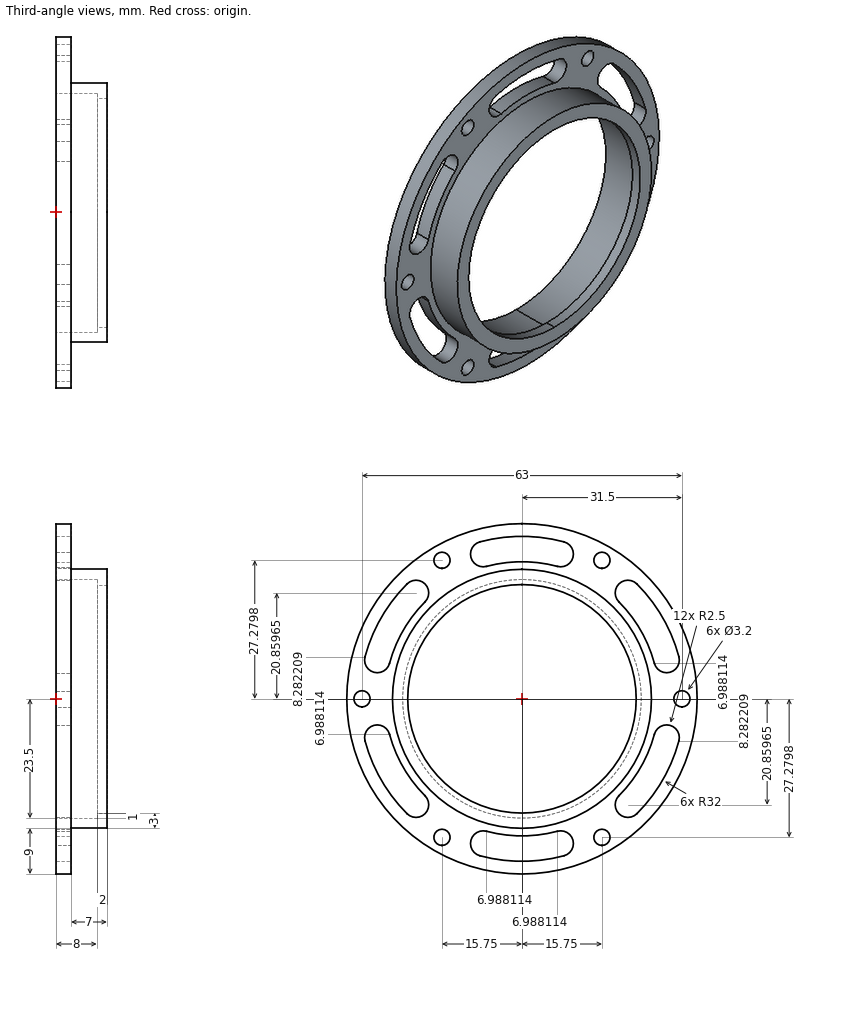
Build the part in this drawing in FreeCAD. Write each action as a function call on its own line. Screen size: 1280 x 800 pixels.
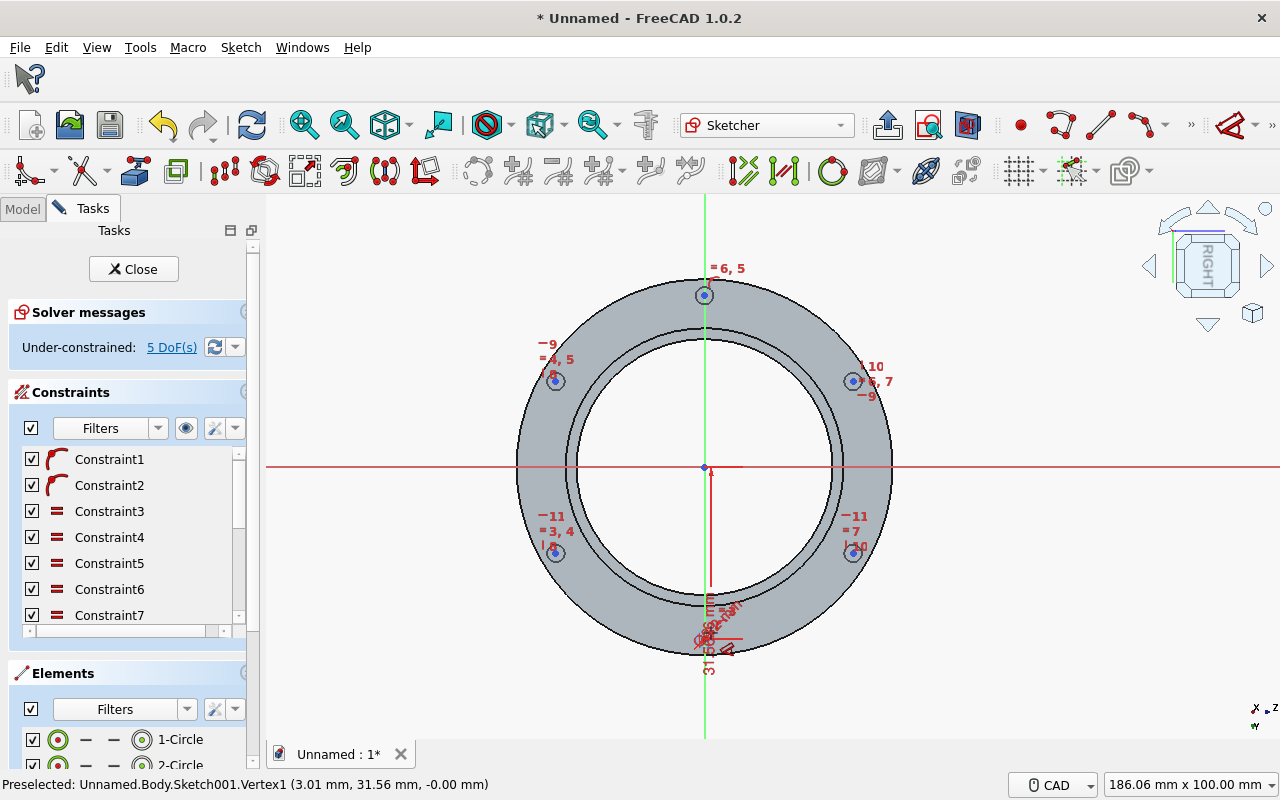
click(705, 296)
click(739, 388)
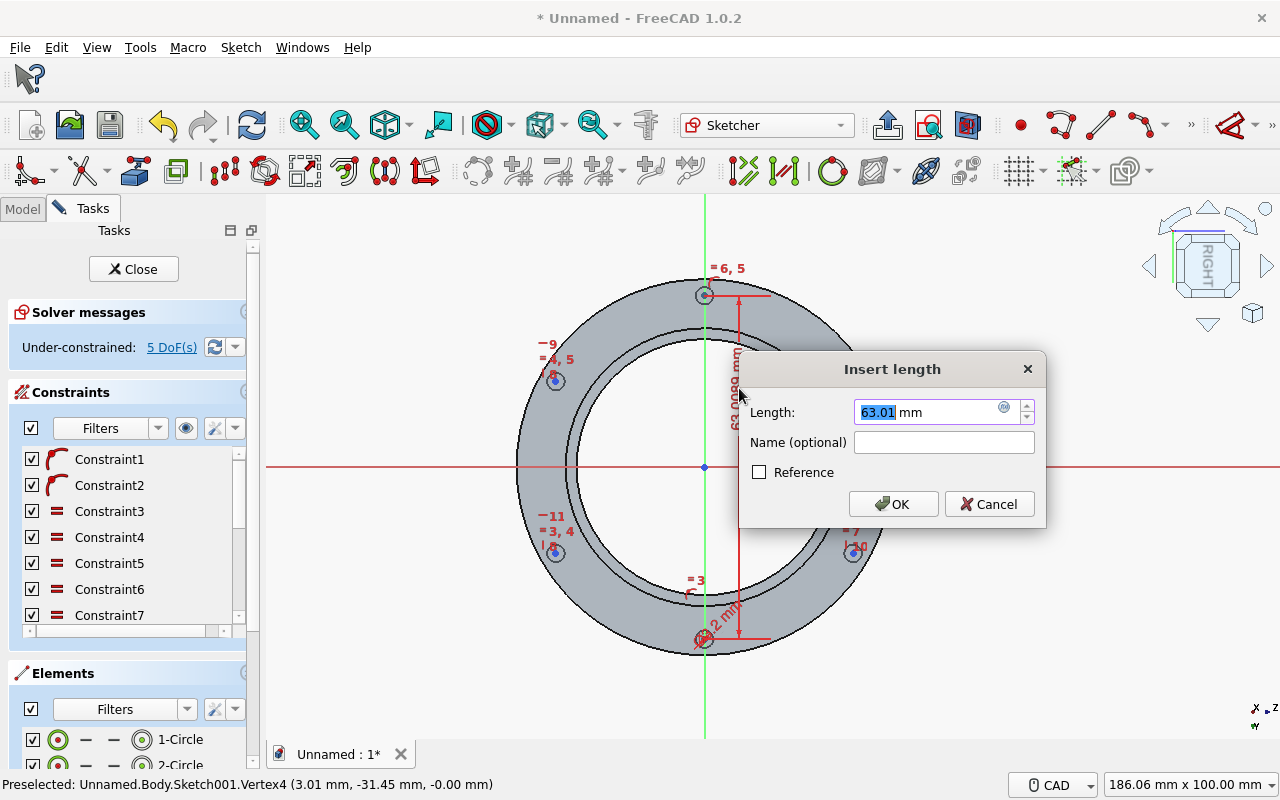
text(63)
key(Return)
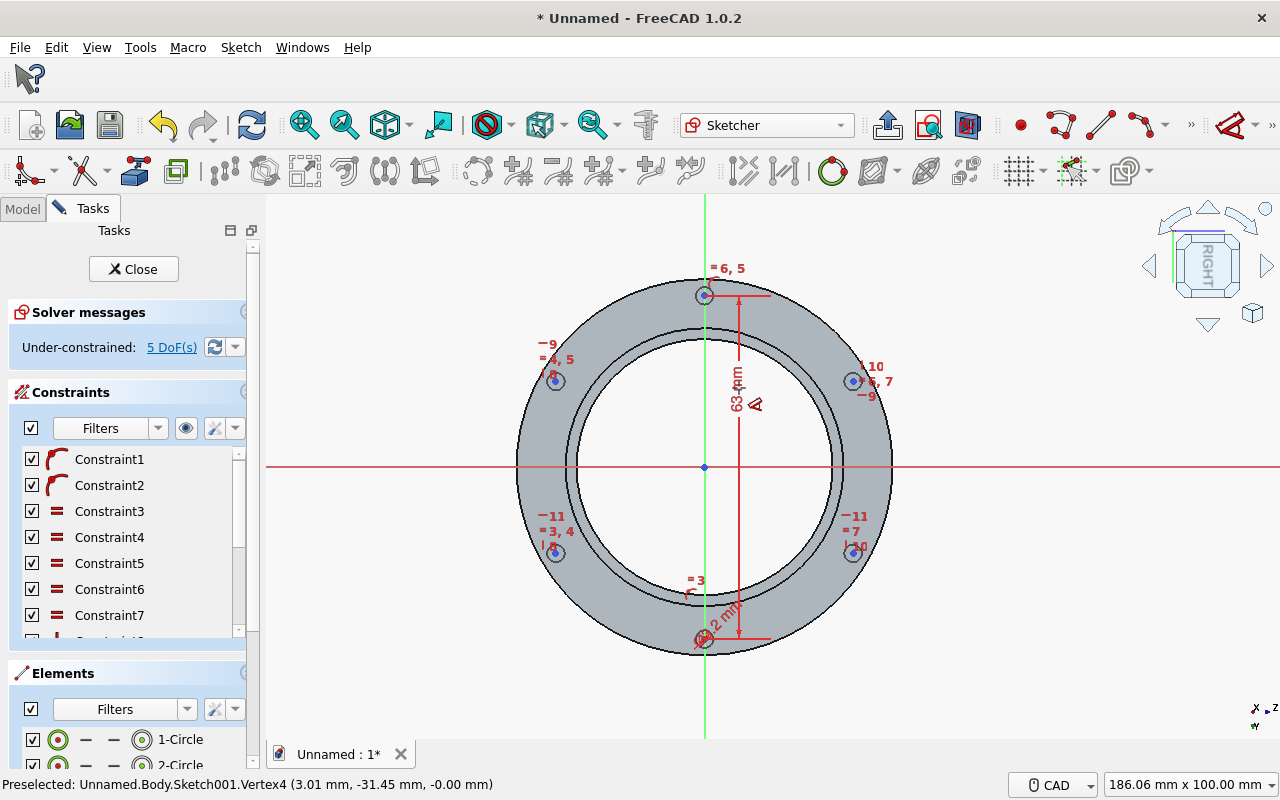
click(705, 639)
click(739, 553)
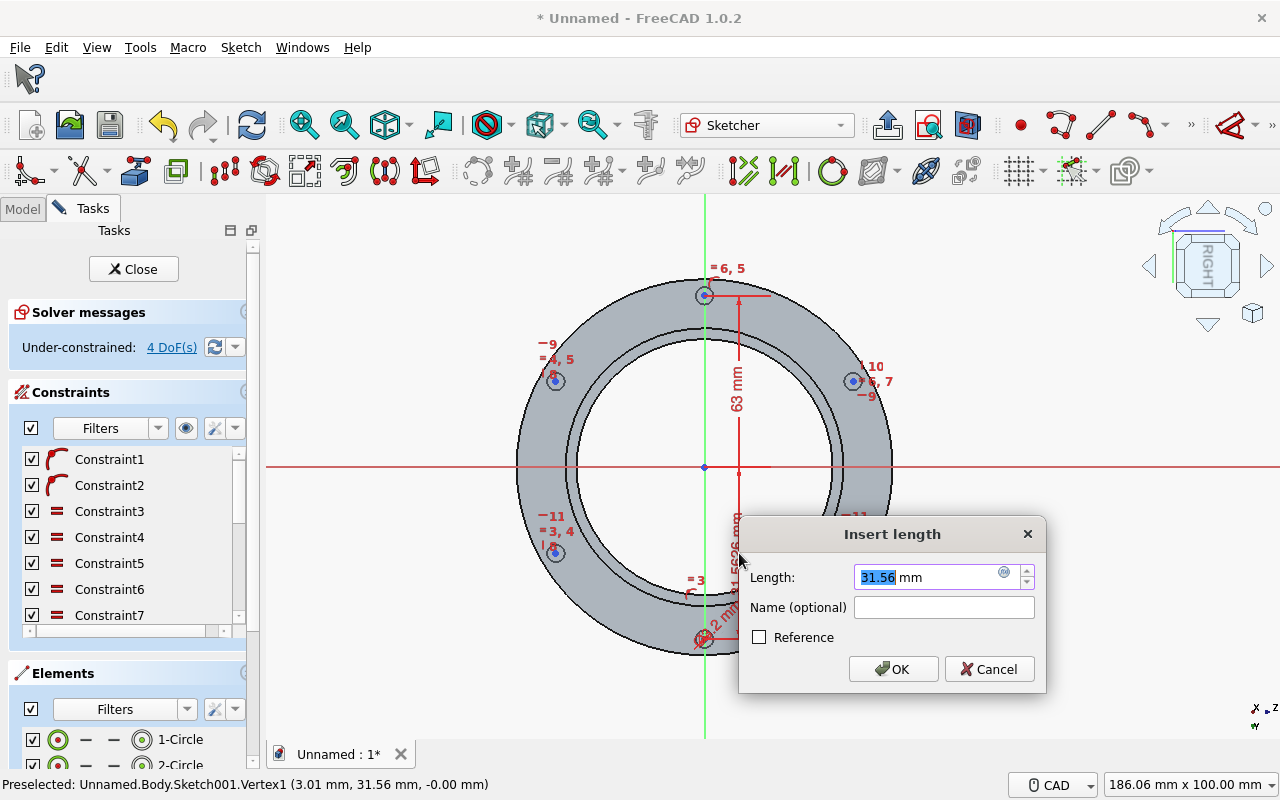
text(31.5)
key(Return)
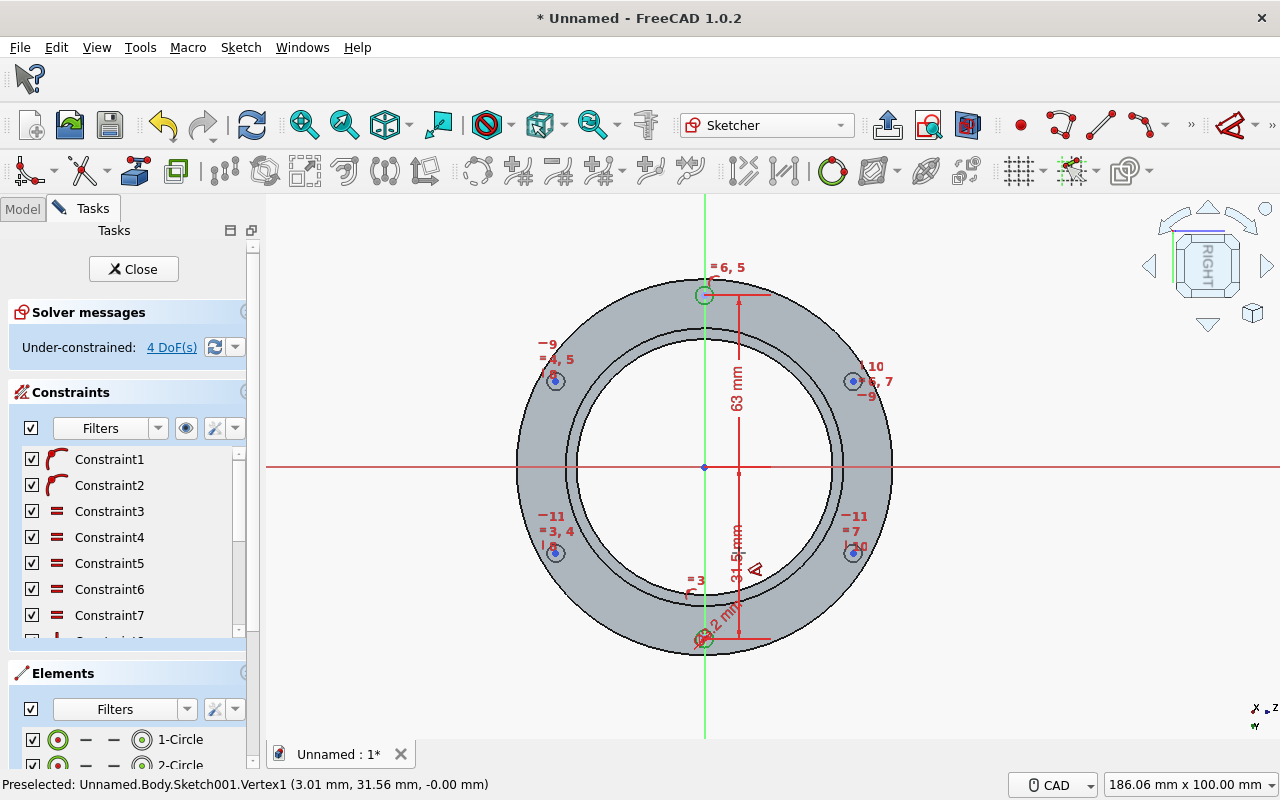
click(556, 553)
click(522, 510)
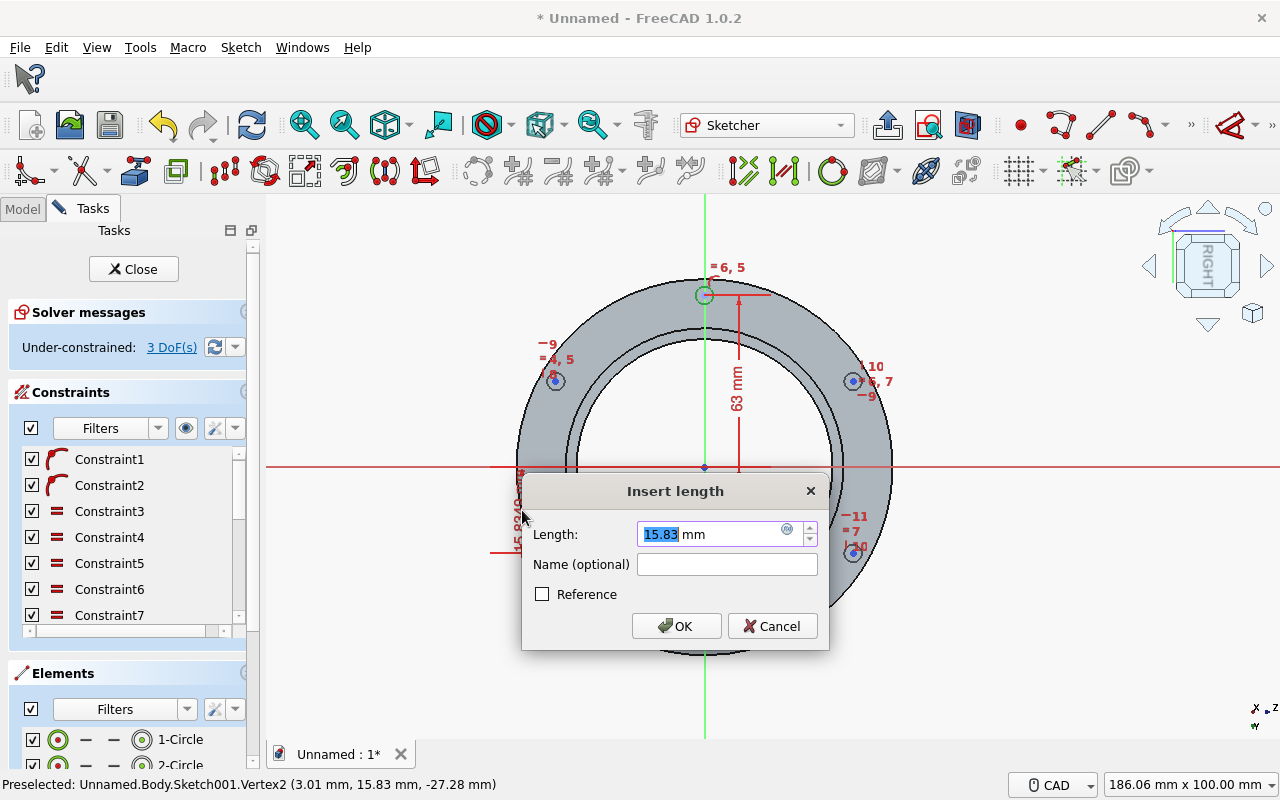
text(15.75)
key(Return)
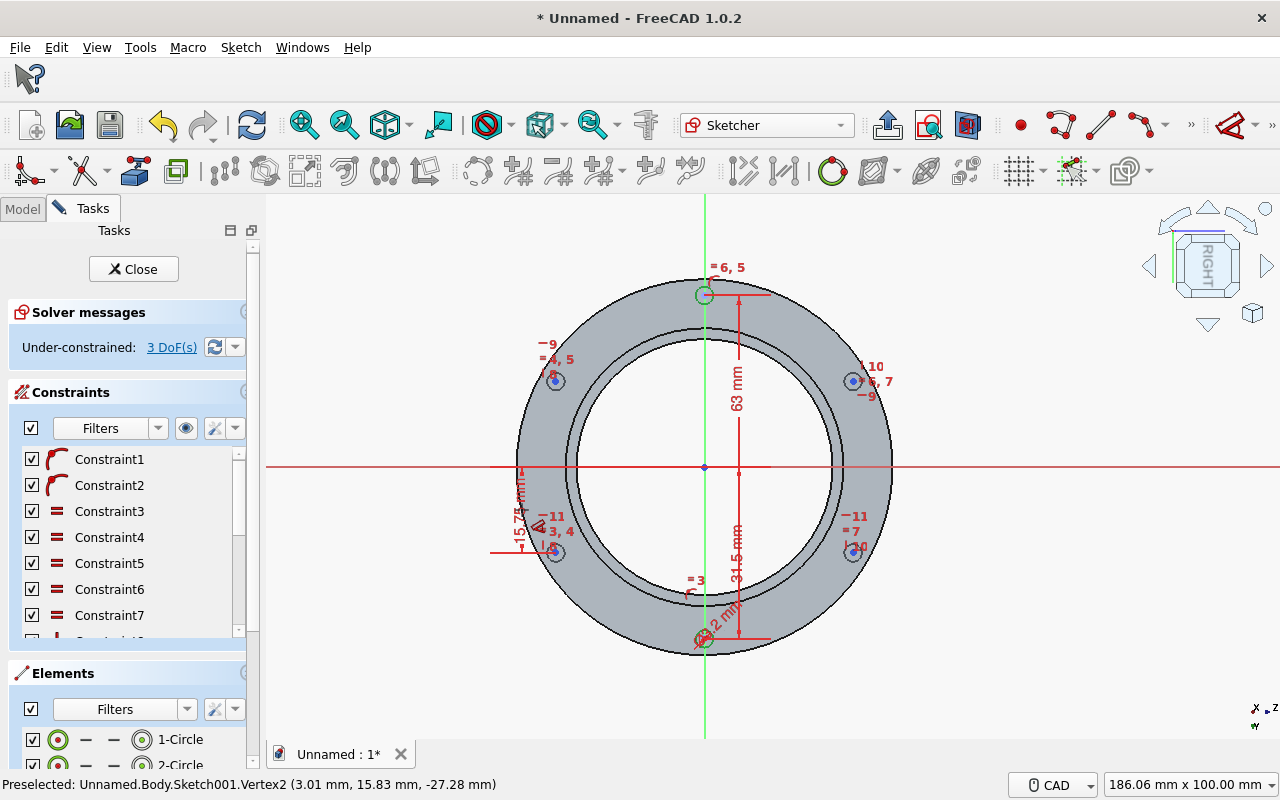
click(556, 382)
click(522, 424)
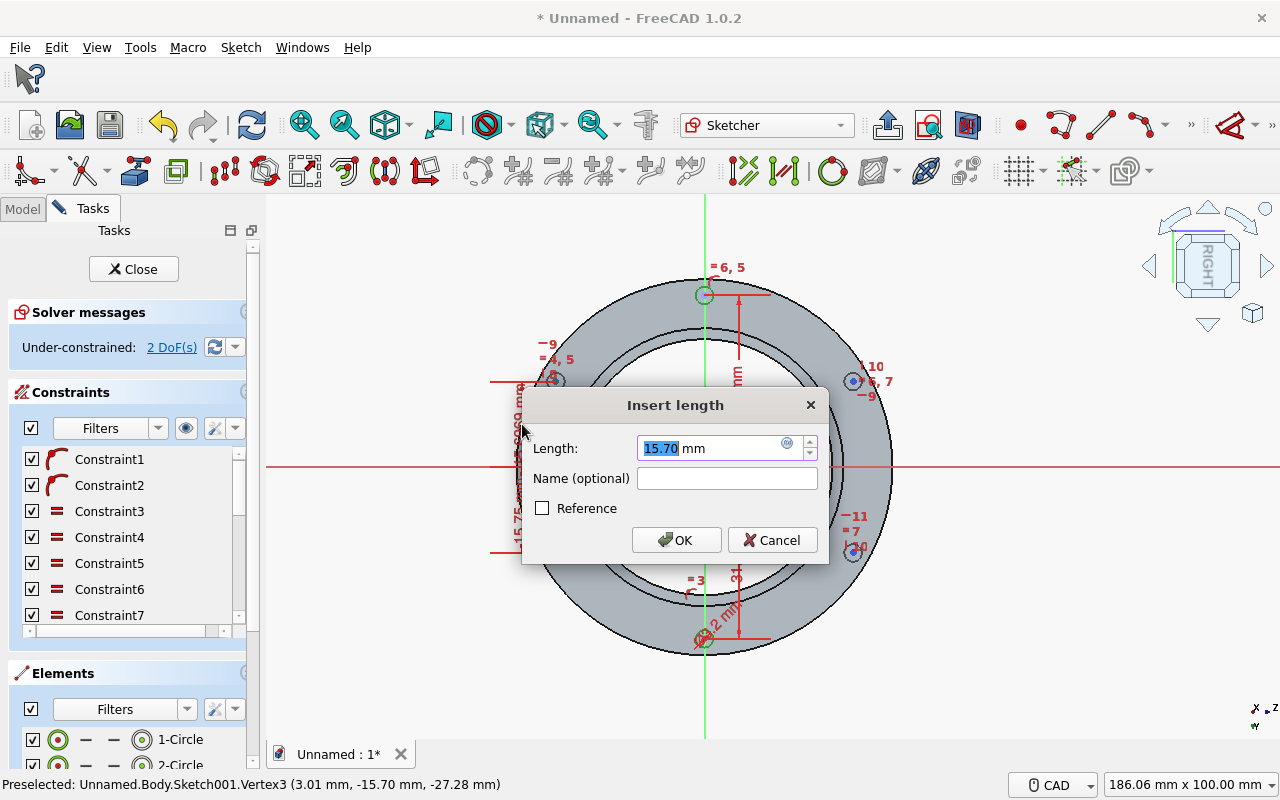
text(15.75)
key(Return)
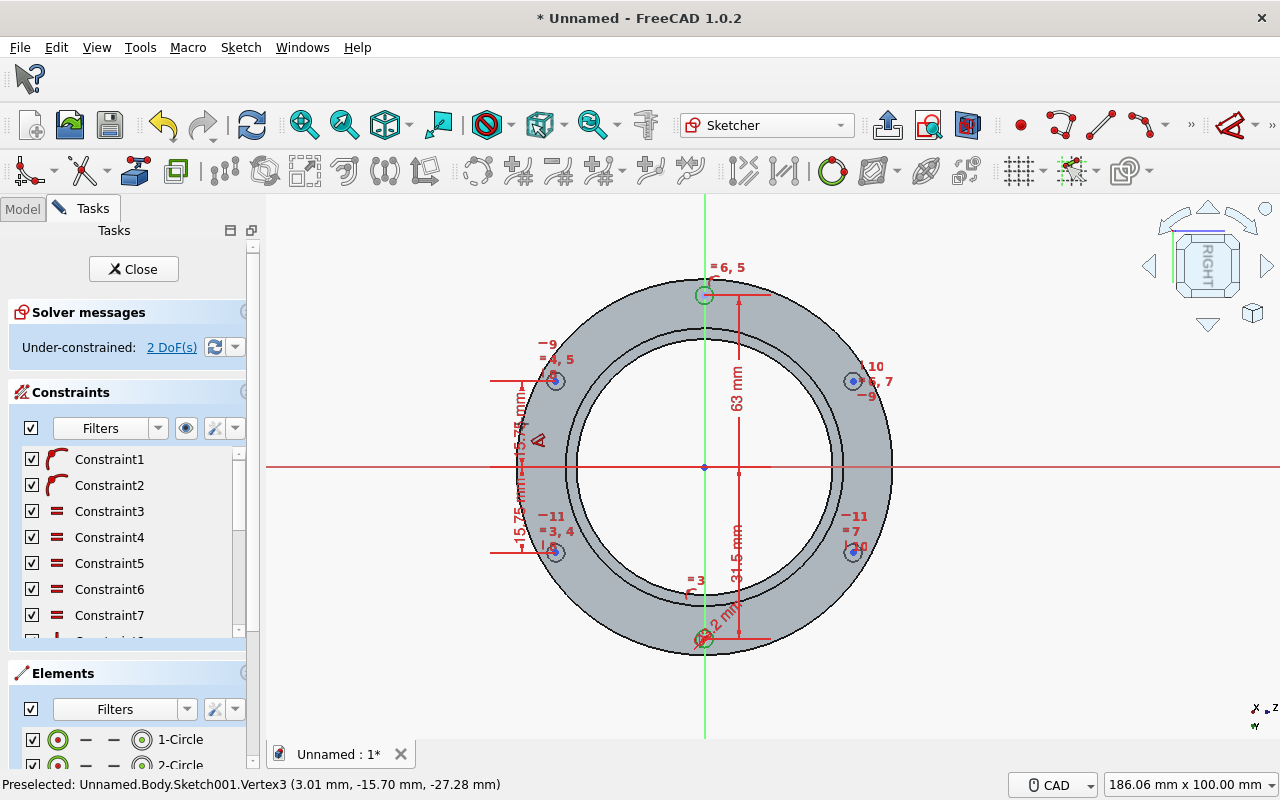
click(556, 553)
click(630, 587)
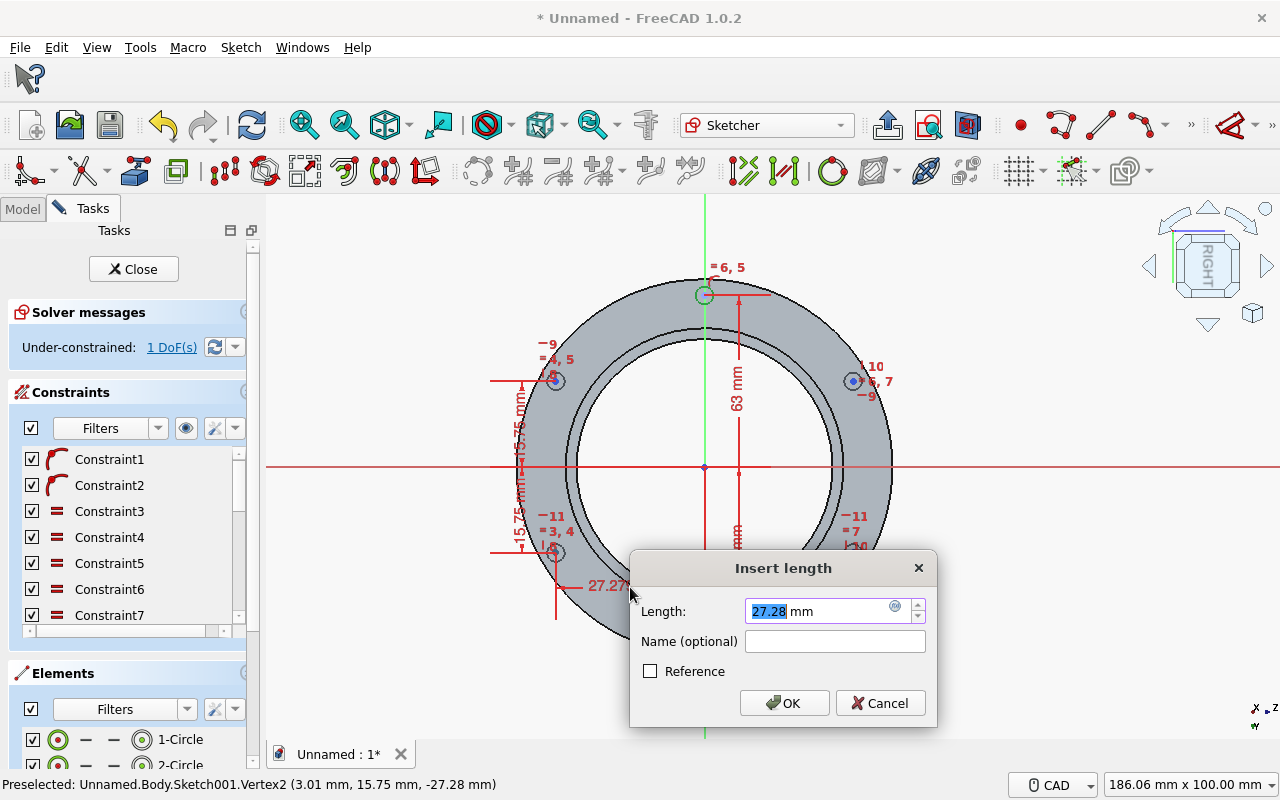
text(27.2798)
key(Return)